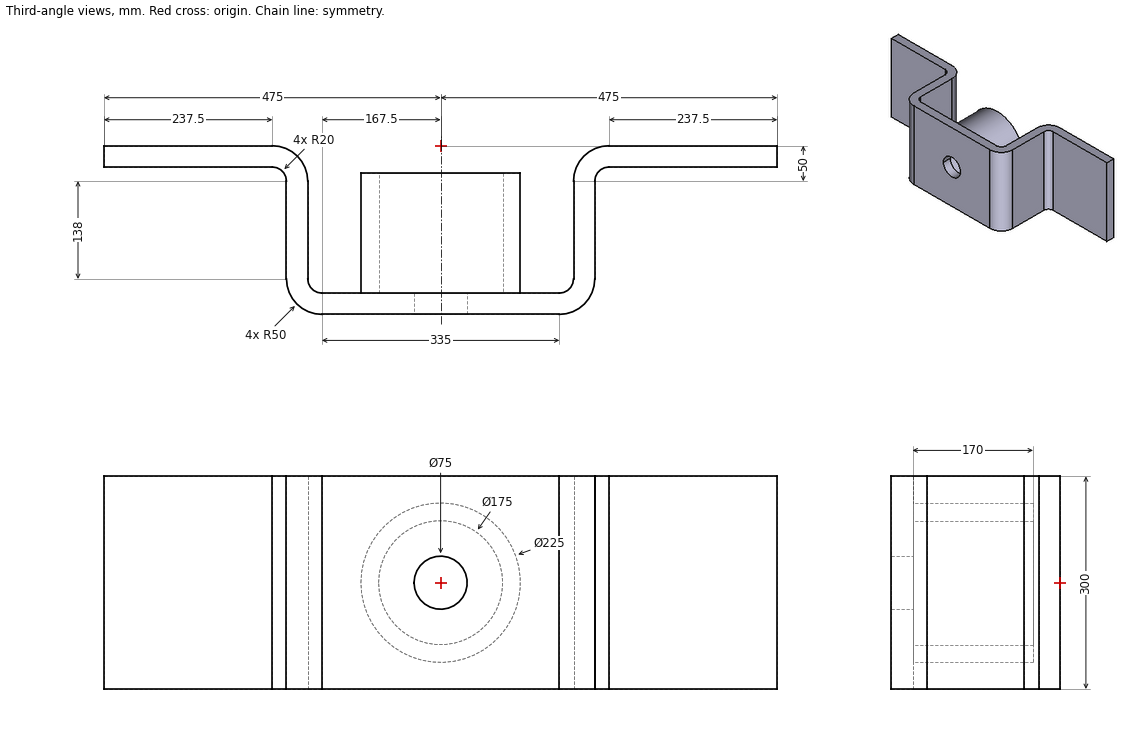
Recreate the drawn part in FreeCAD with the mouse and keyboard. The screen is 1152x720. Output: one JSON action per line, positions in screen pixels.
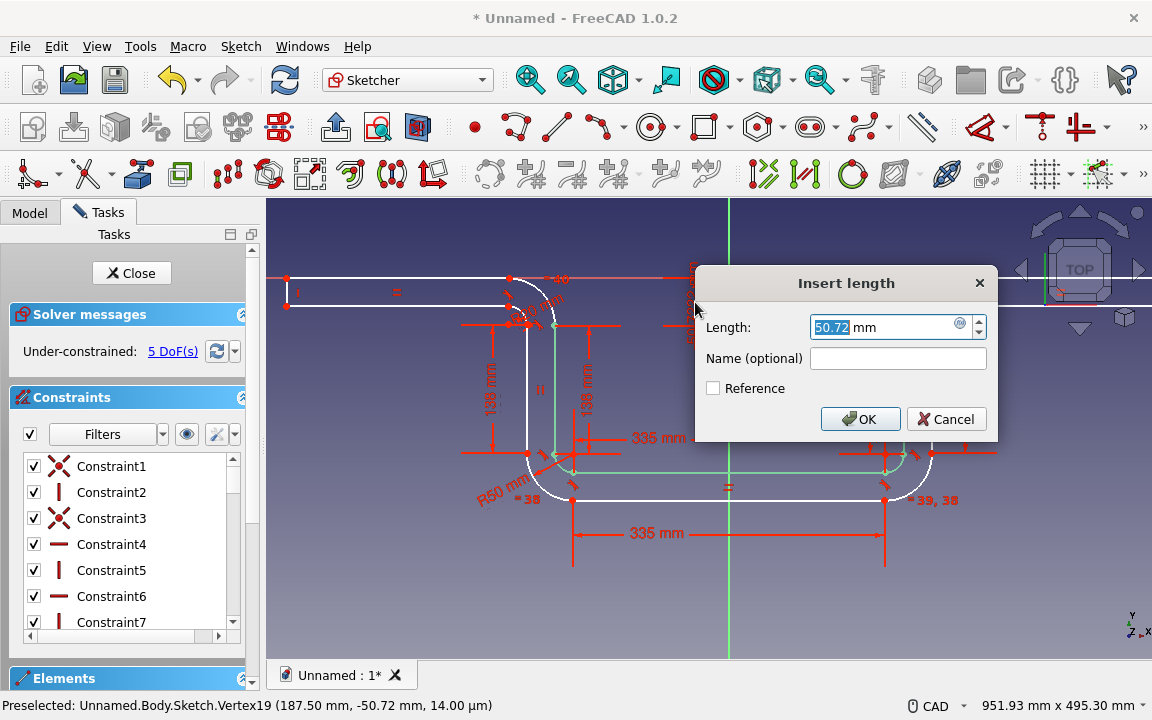
{"action": "type", "text": "50"}
{"action": "key", "text": "Return"}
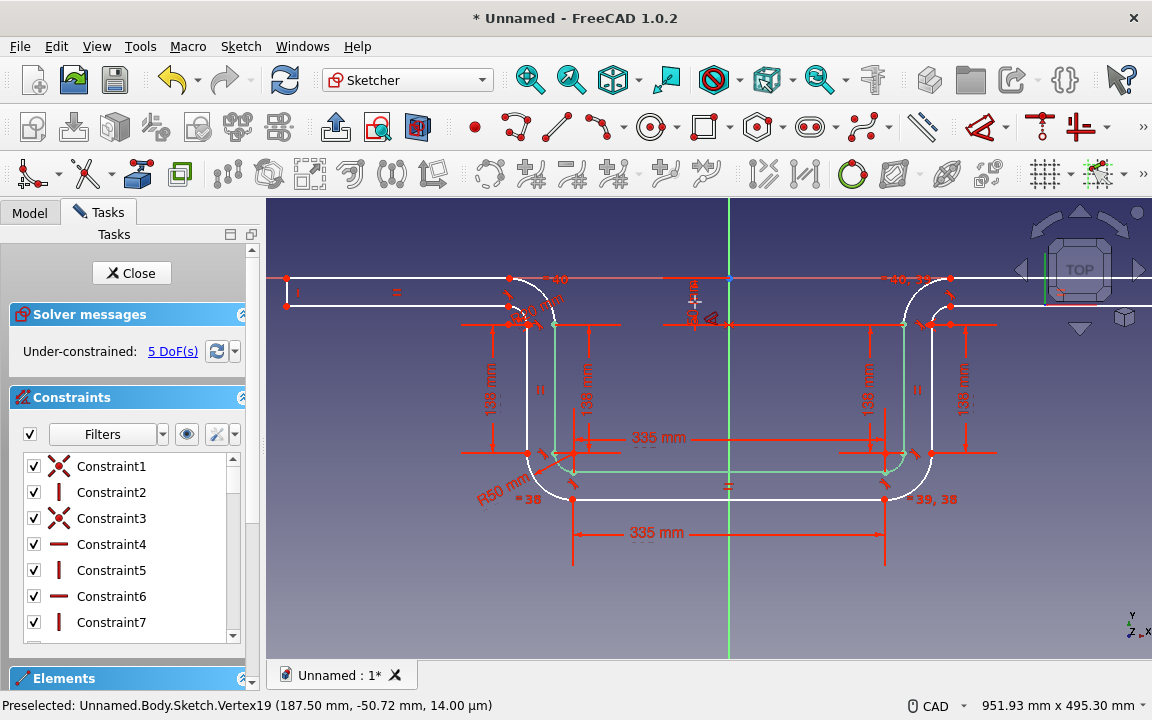
{"action": "scroll", "coordinate": [532, 476], "scroll_direction": "down", "scroll_amount": 3}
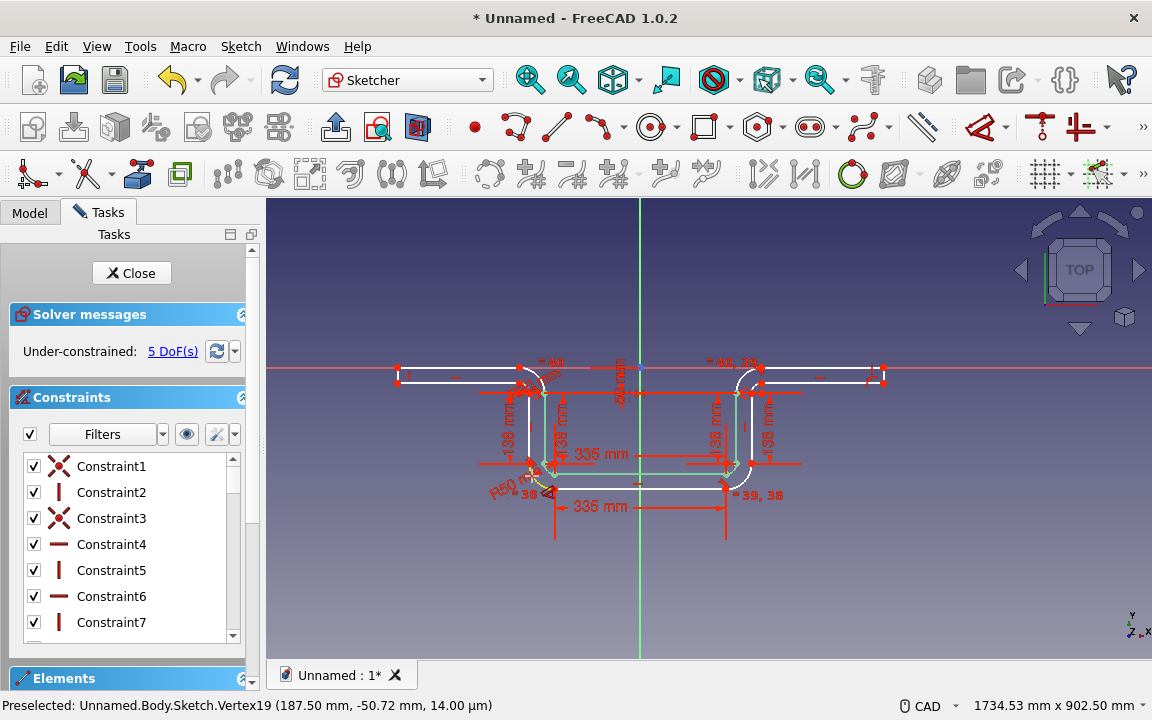
{"action": "left_click", "coordinate": [398, 368]}
{"action": "left_click", "coordinate": [519, 334]}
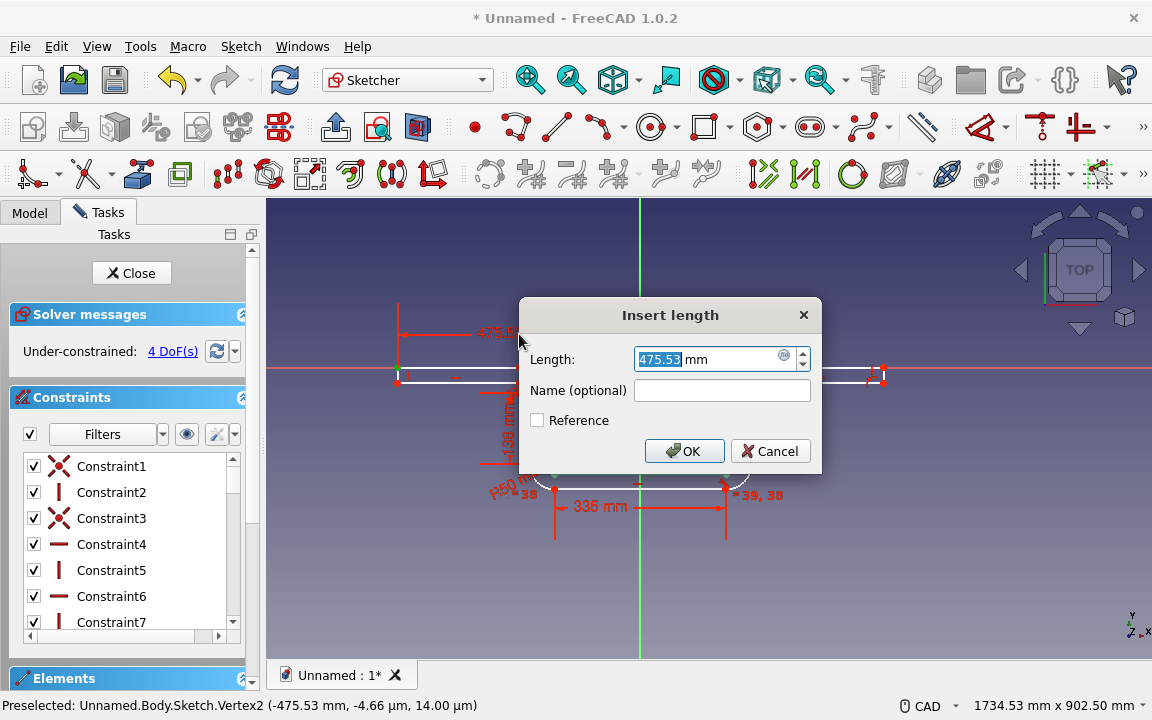
{"action": "type", "text": "475"}
{"action": "key", "text": "Return"}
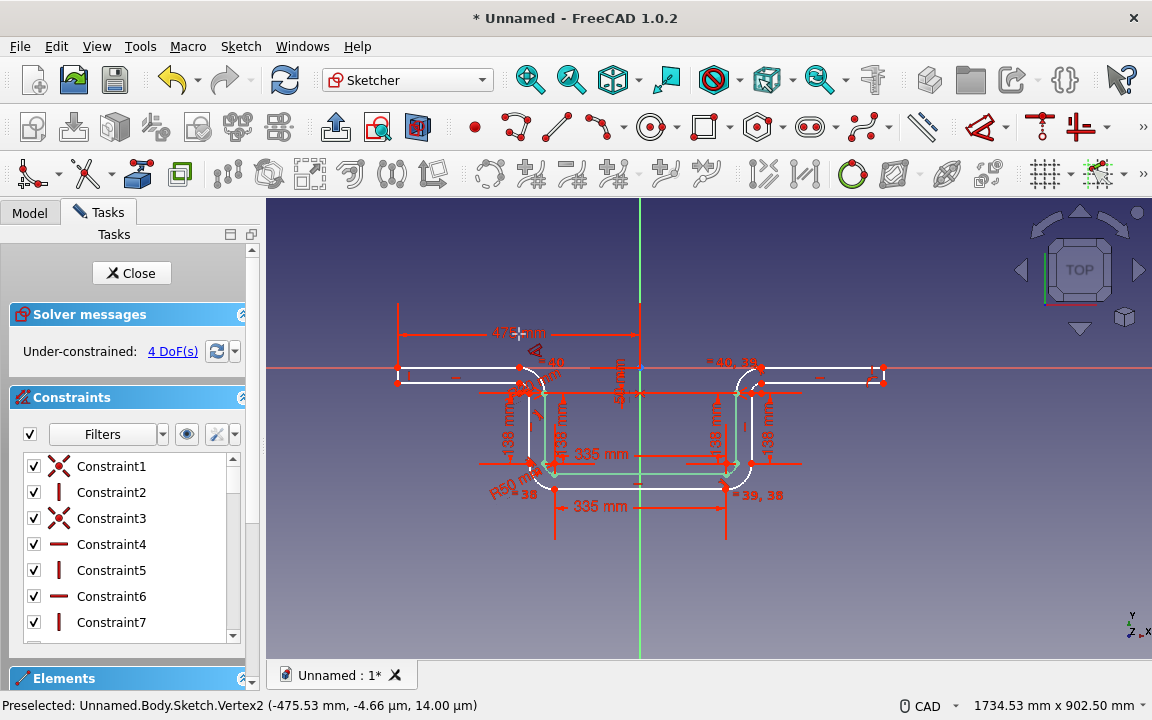
{"action": "left_click", "coordinate": [884, 383]}
{"action": "left_click", "coordinate": [762, 334]}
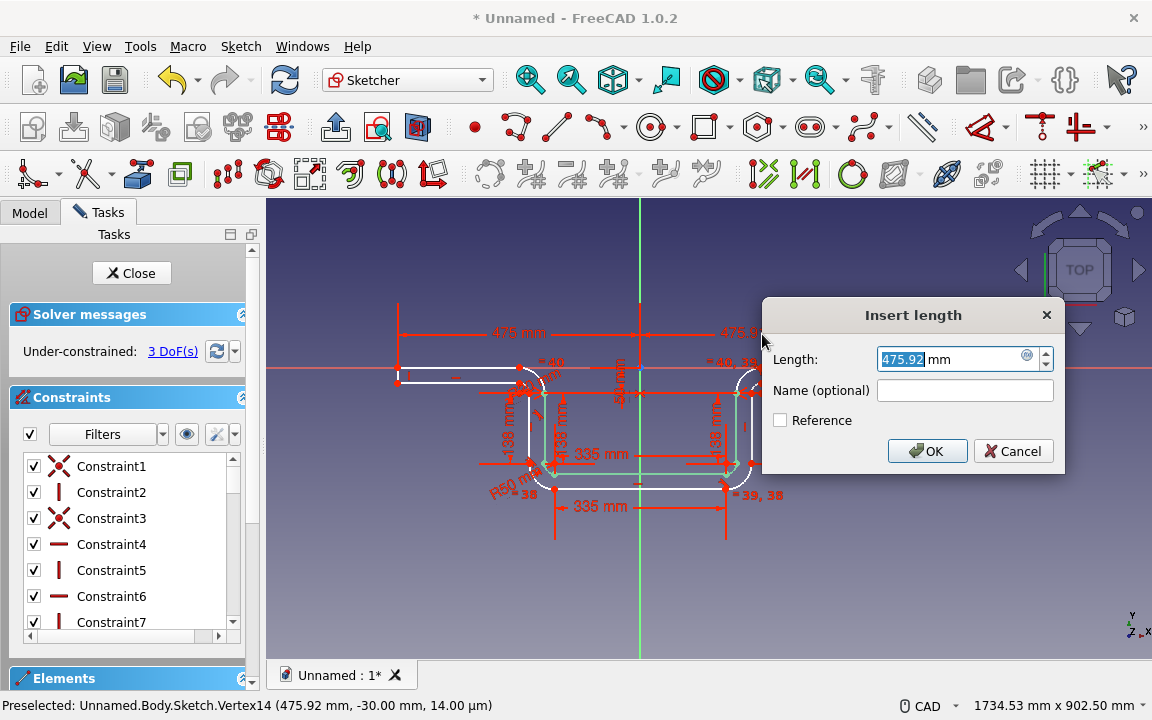
{"action": "type", "text": "475"}
{"action": "key", "text": "Return"}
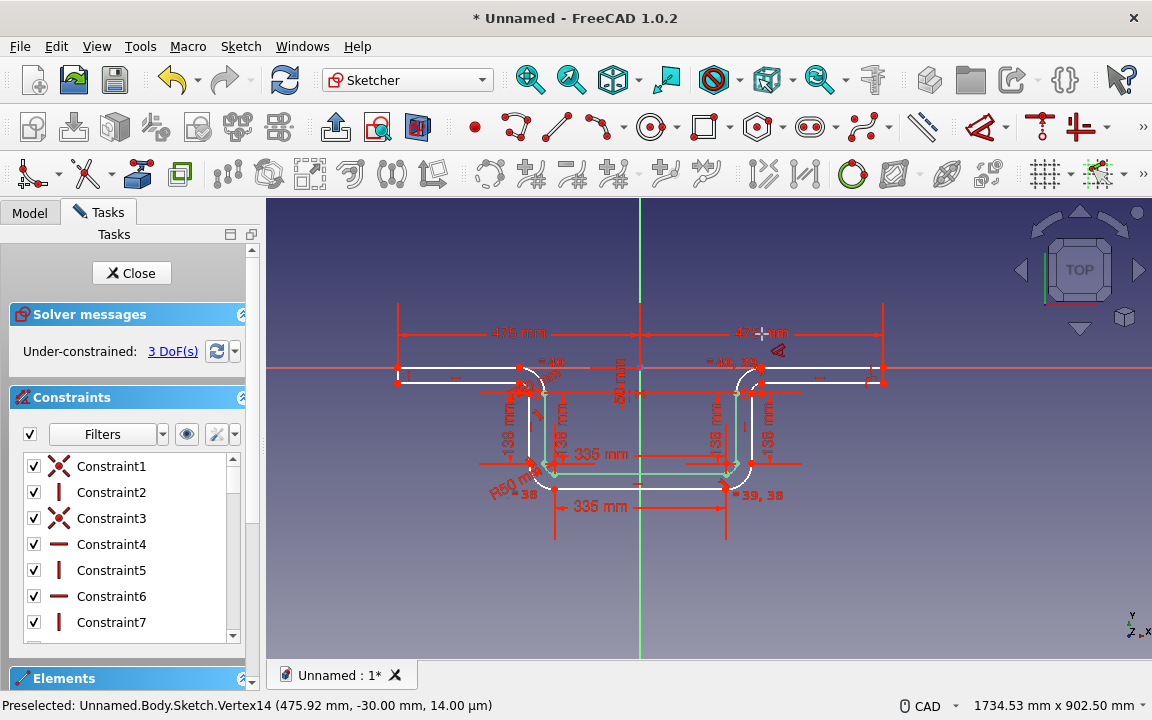
{"action": "left_click", "coordinate": [483, 368]}
{"action": "left_click", "coordinate": [431, 334]}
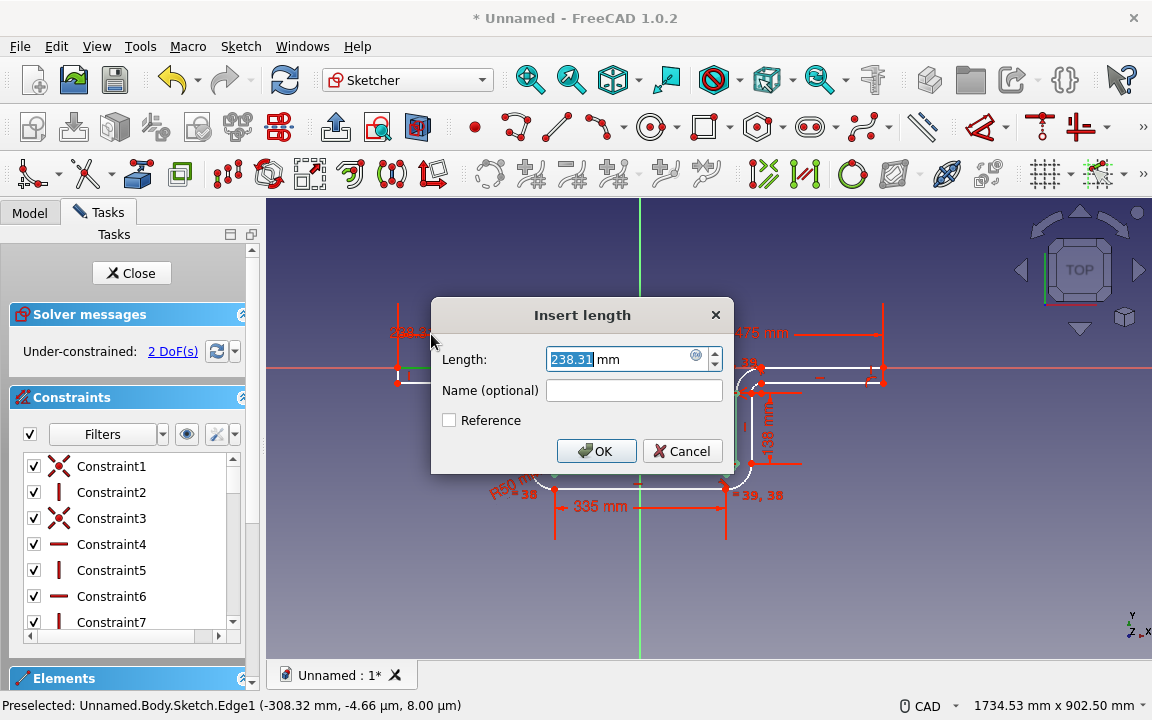
{"action": "type", "text": "237.5"}
{"action": "key", "text": "Return"}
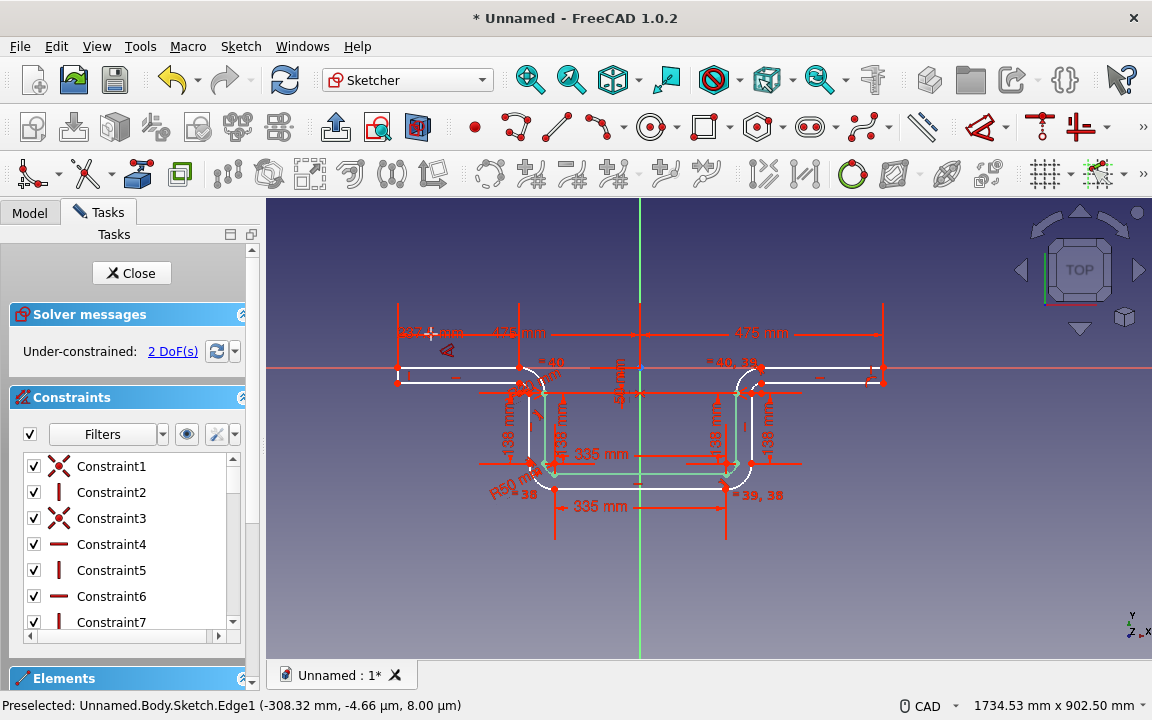
{"action": "left_click", "coordinate": [847, 368]}
{"action": "left_click", "coordinate": [850, 334]}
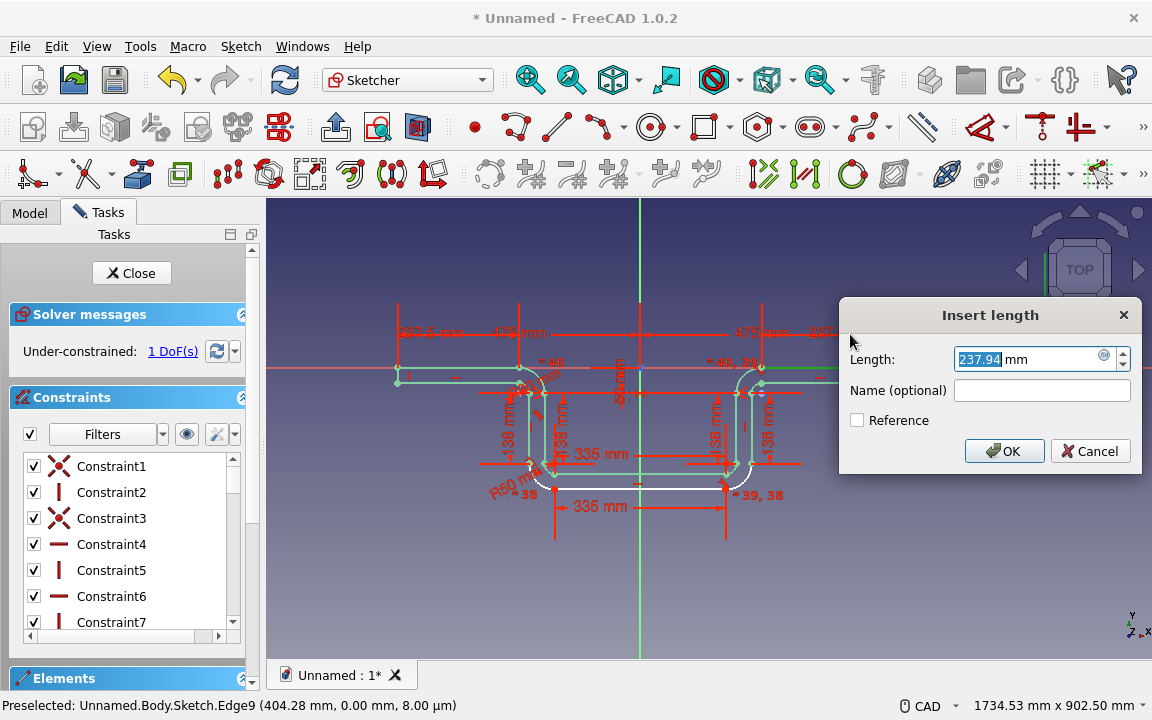
{"action": "type", "text": "237.5"}
{"action": "key", "text": "Return"}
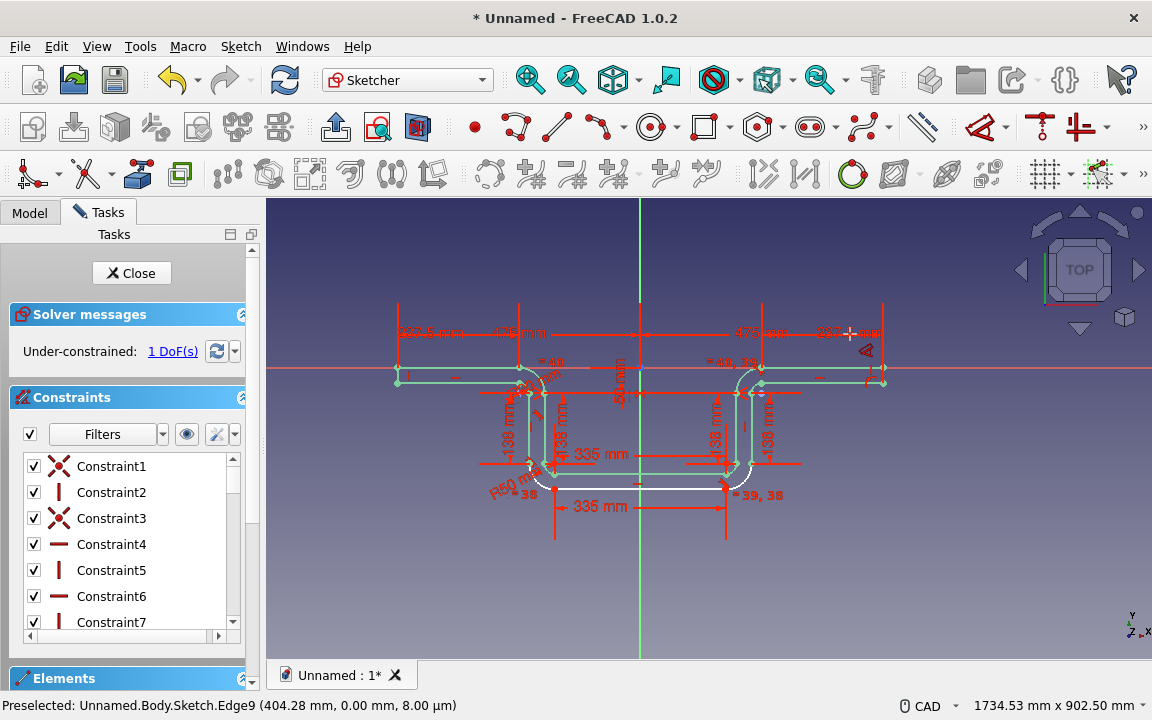
{"action": "left_click", "coordinate": [555, 489]}
{"action": "left_click", "coordinate": [598, 334]}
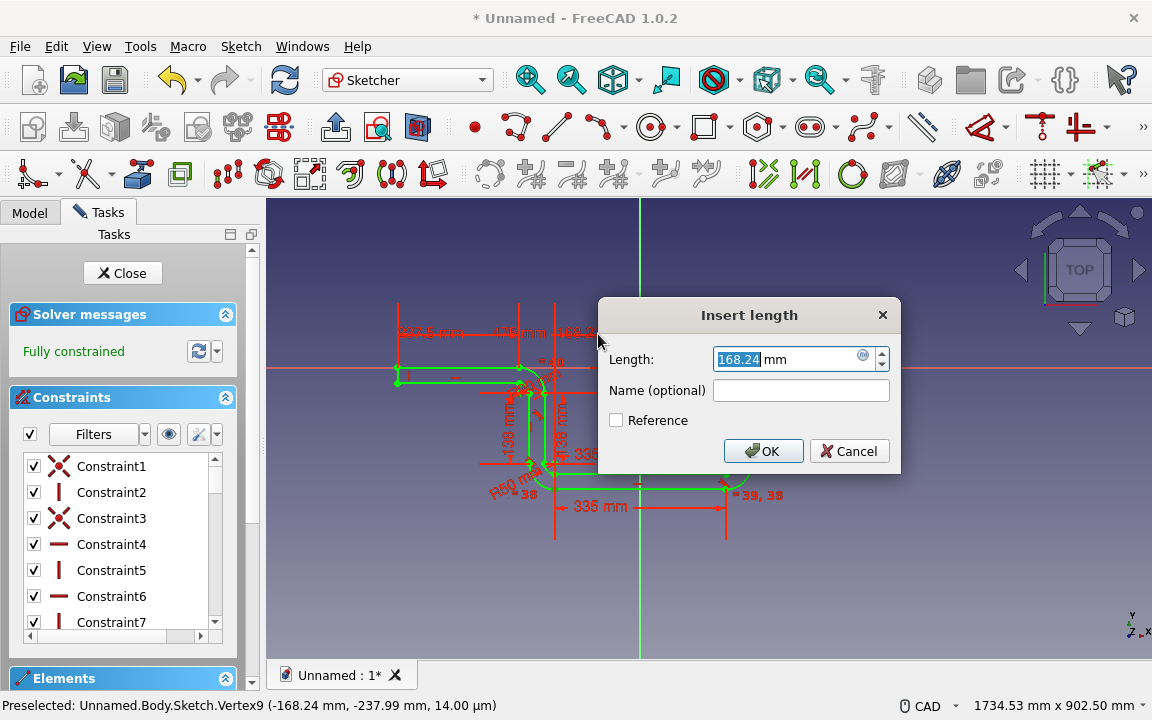
{"action": "type", "text": "167.5"}
{"action": "key", "text": "Return"}
{"action": "key", "text": "Escape"}